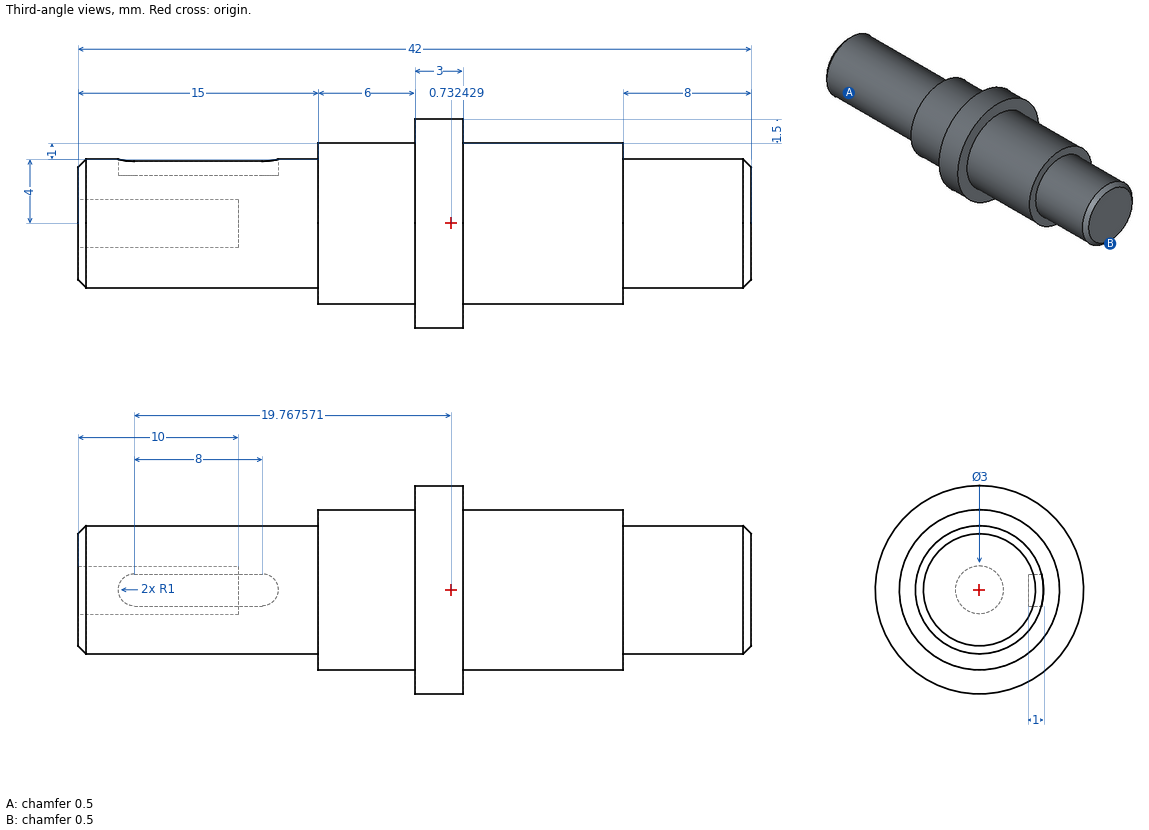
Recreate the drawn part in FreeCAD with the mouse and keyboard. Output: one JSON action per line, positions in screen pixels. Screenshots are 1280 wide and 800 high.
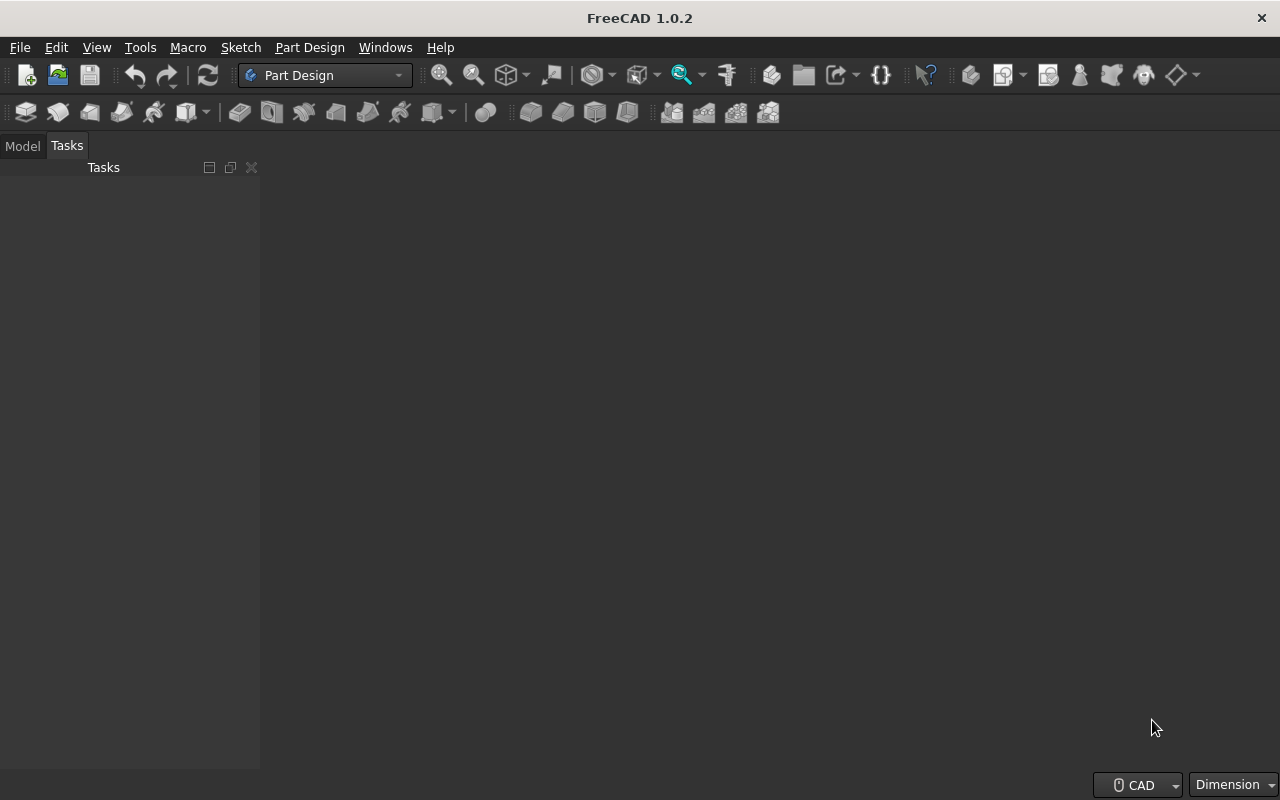
{"action": "left_click", "coordinate": [26, 76]}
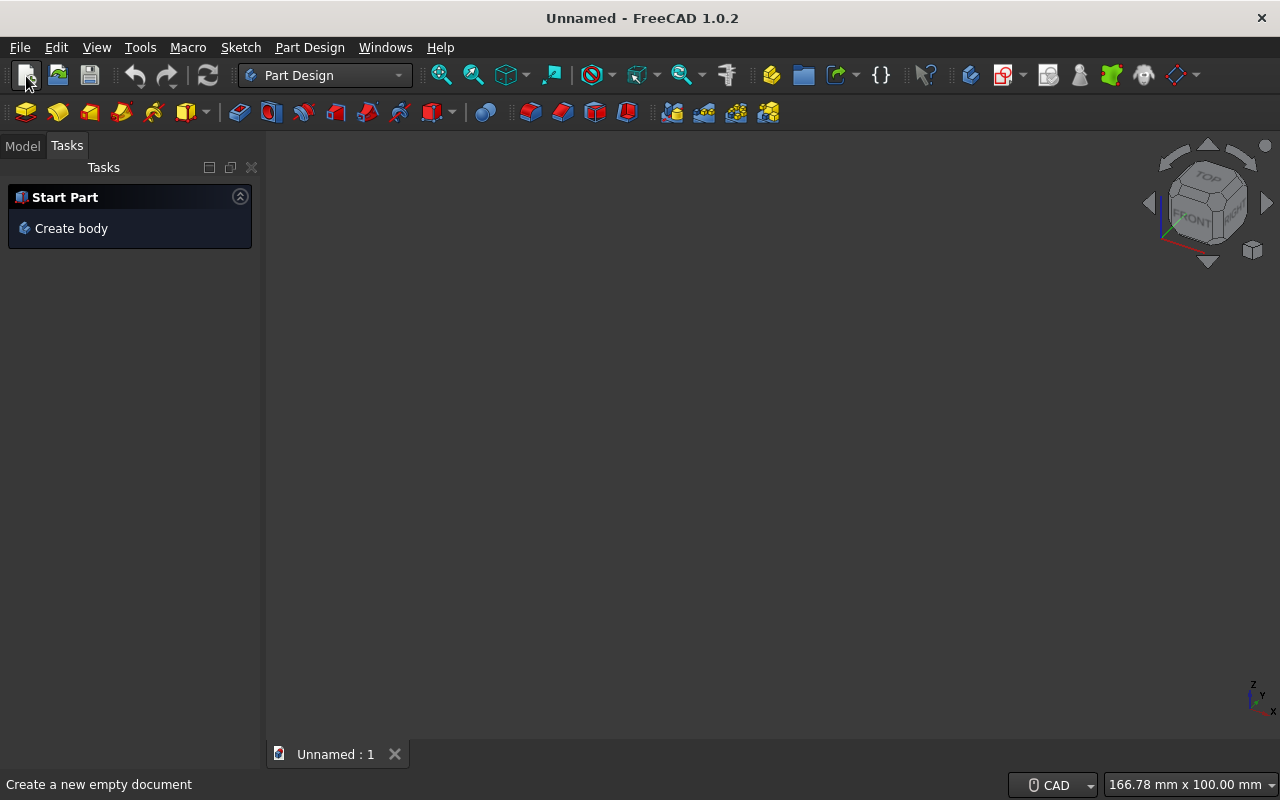
{"action": "left_click", "coordinate": [1004, 76]}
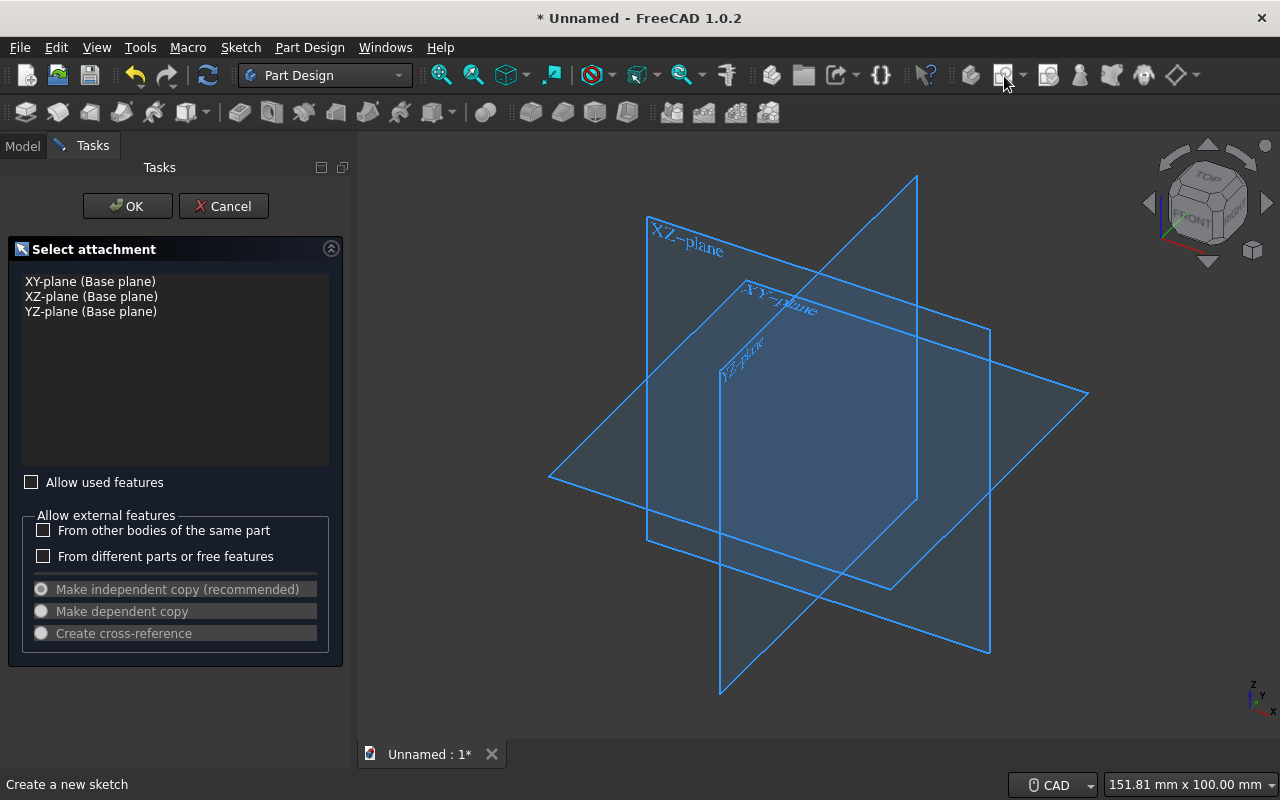
{"action": "left_click", "coordinate": [82, 282]}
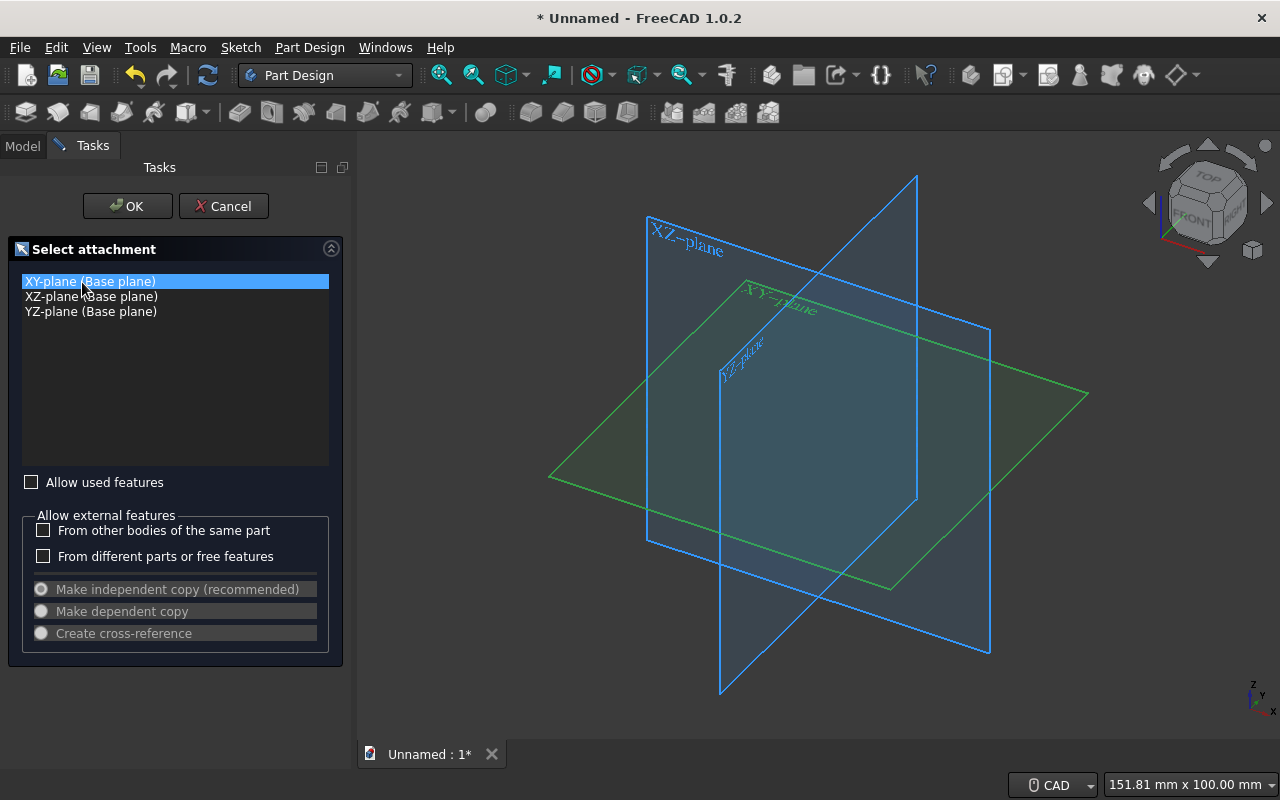
{"action": "left_click", "coordinate": [128, 206]}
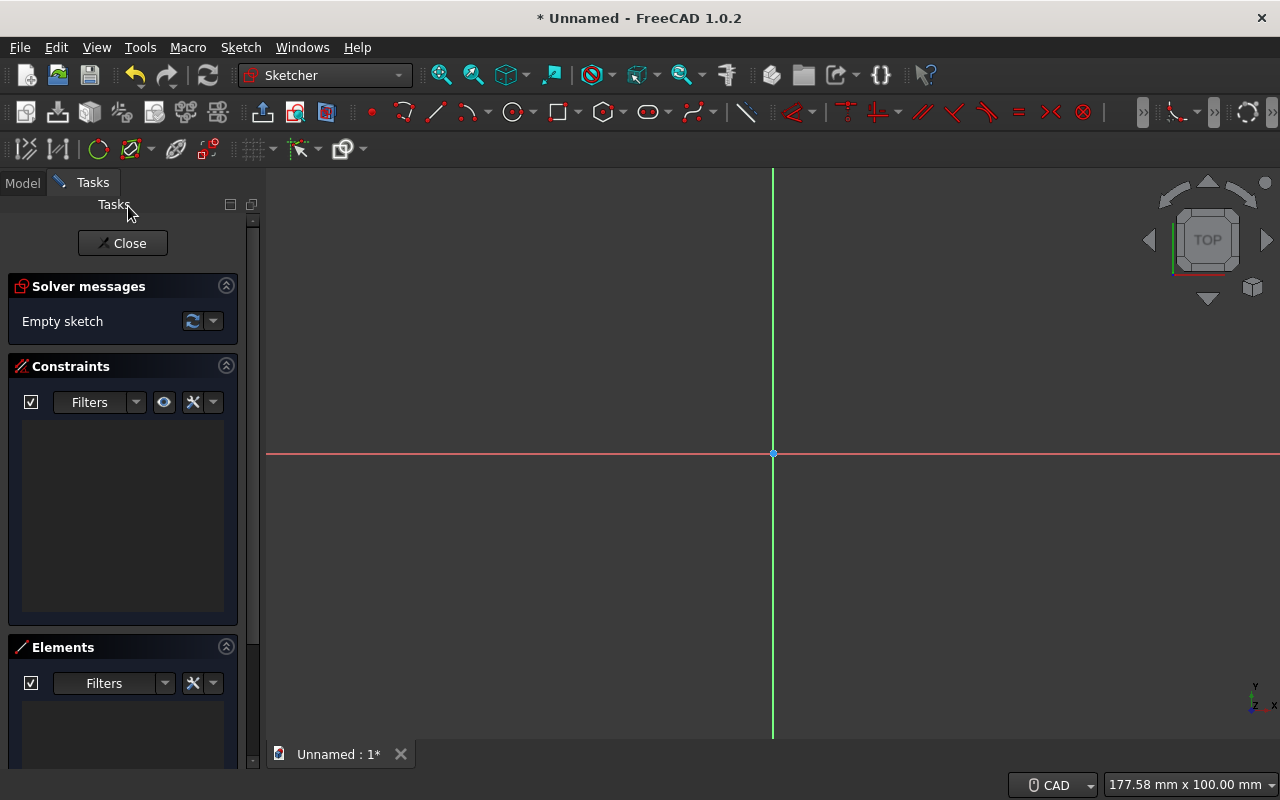
{"action": "scroll", "coordinate": [805, 420], "scroll_direction": "up", "scroll_amount": 4}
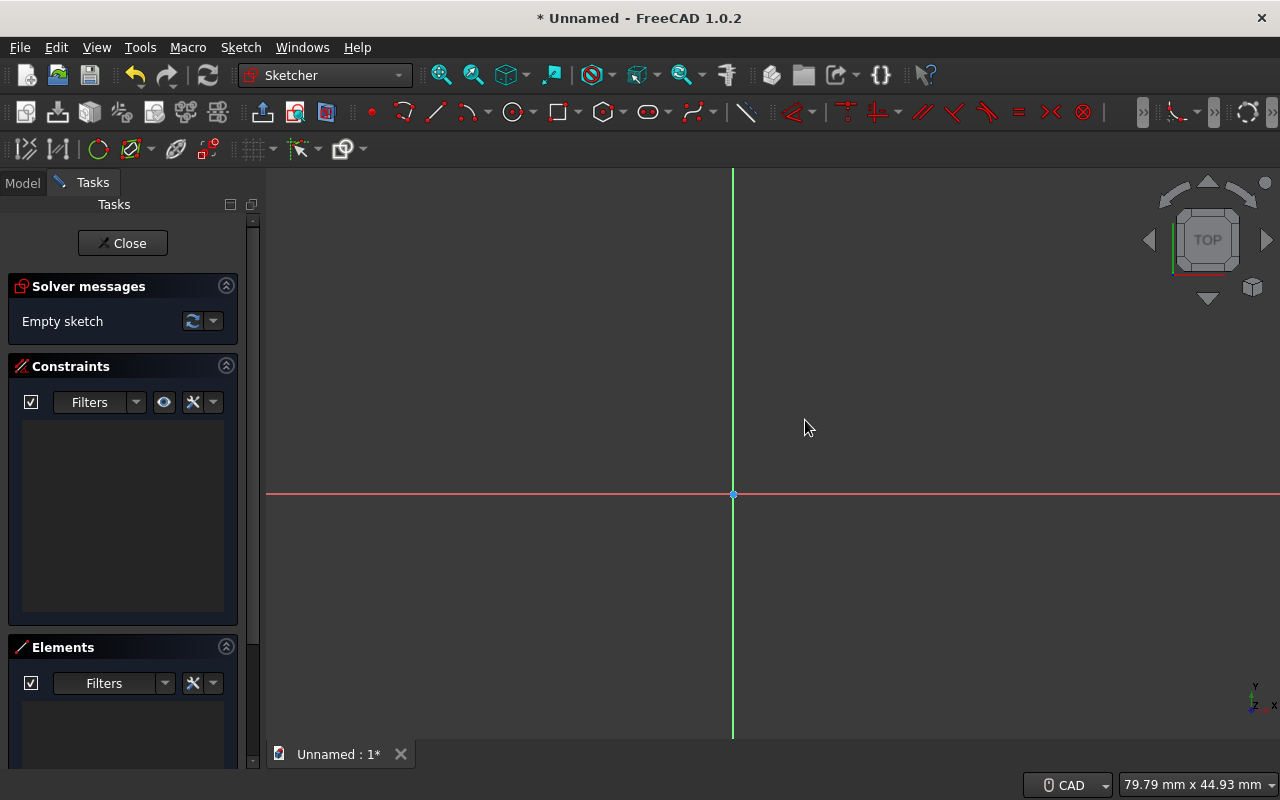
{"action": "left_click", "coordinate": [404, 112]}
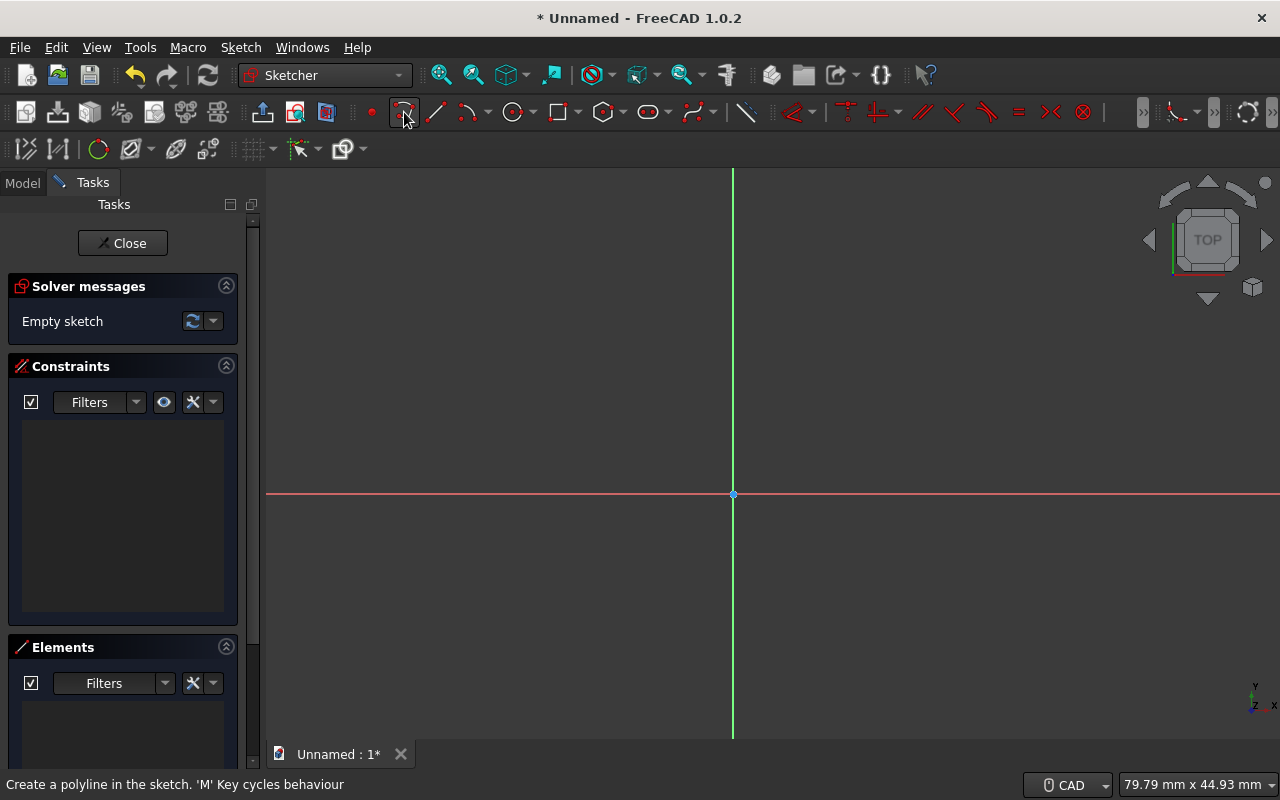
{"action": "scroll", "coordinate": [742, 430], "scroll_direction": "up", "scroll_amount": 3}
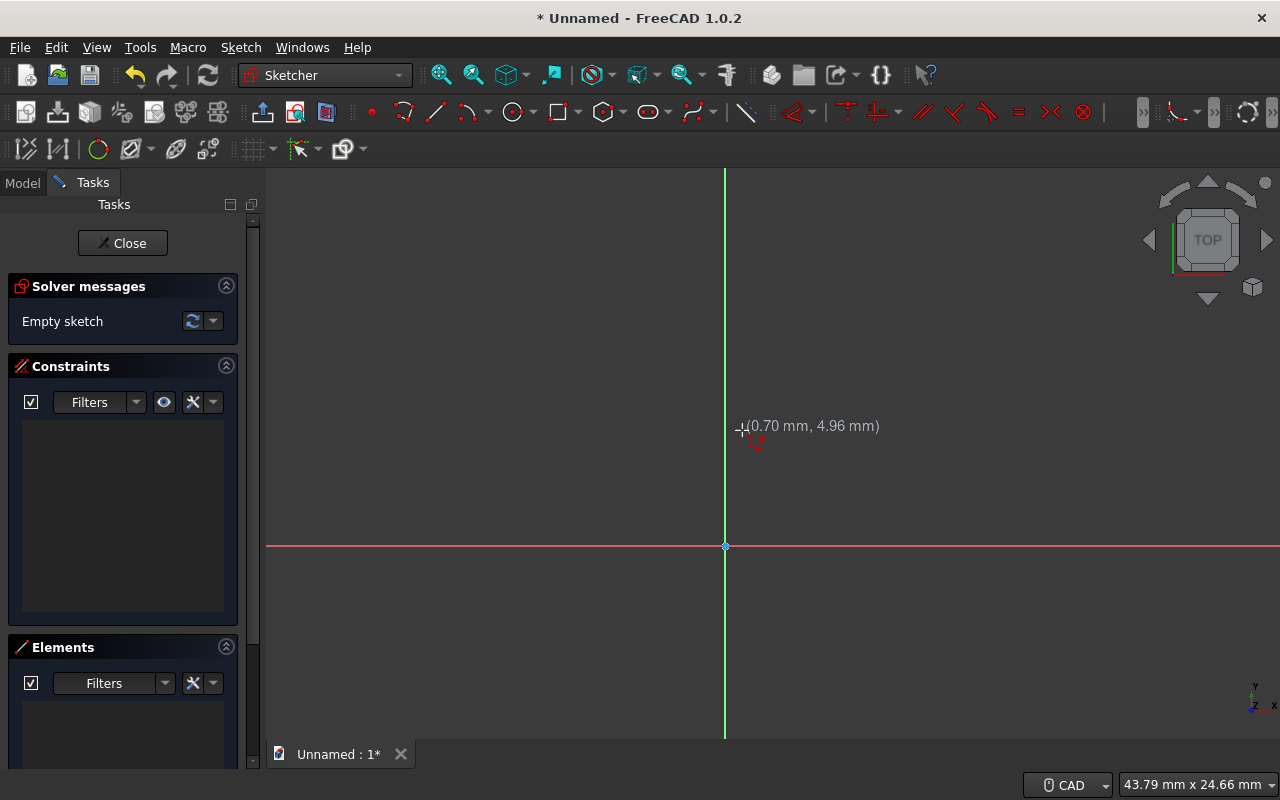
{"action": "left_click", "coordinate": [742, 430]}
{"action": "left_click", "coordinate": [742, 396]}
{"action": "left_click", "coordinate": [673, 396]}
{"action": "left_click", "coordinate": [673, 430]}
{"action": "left_click", "coordinate": [534, 430]}
{"action": "left_click", "coordinate": [534, 454]}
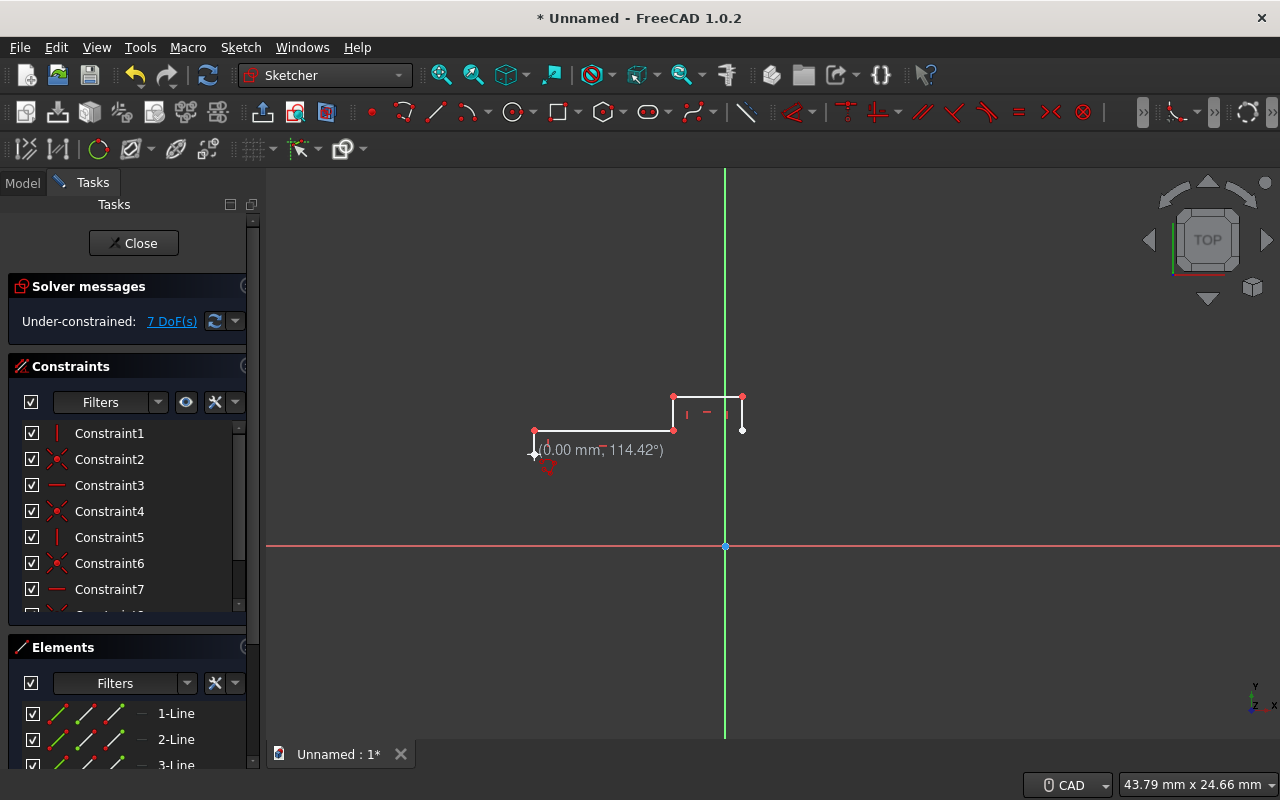
{"action": "scroll", "coordinate": [743, 432], "scroll_direction": "down", "scroll_amount": 3}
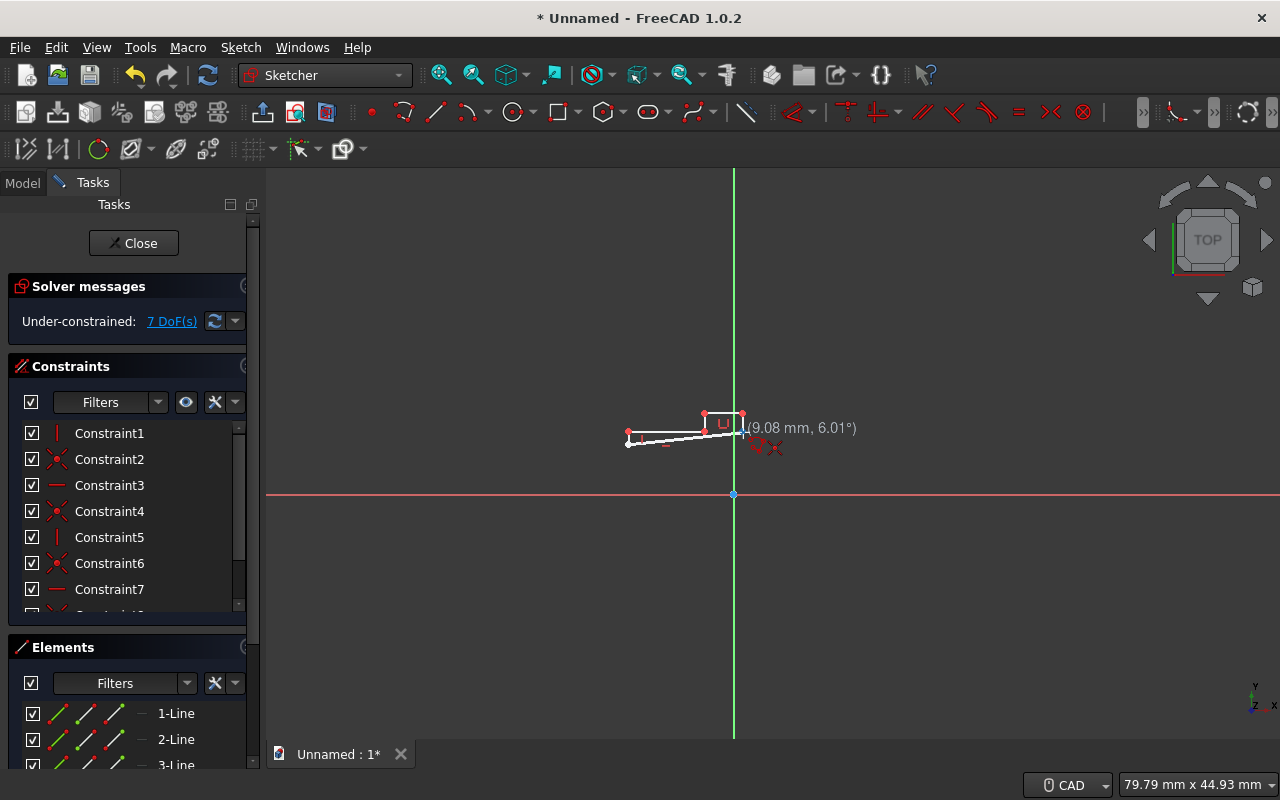
{"action": "left_click", "coordinate": [438, 444]}
{"action": "left_click", "coordinate": [438, 495]}
{"action": "left_click", "coordinate": [972, 486]}
{"action": "left_click", "coordinate": [972, 444]}
{"action": "left_click", "coordinate": [870, 444]}